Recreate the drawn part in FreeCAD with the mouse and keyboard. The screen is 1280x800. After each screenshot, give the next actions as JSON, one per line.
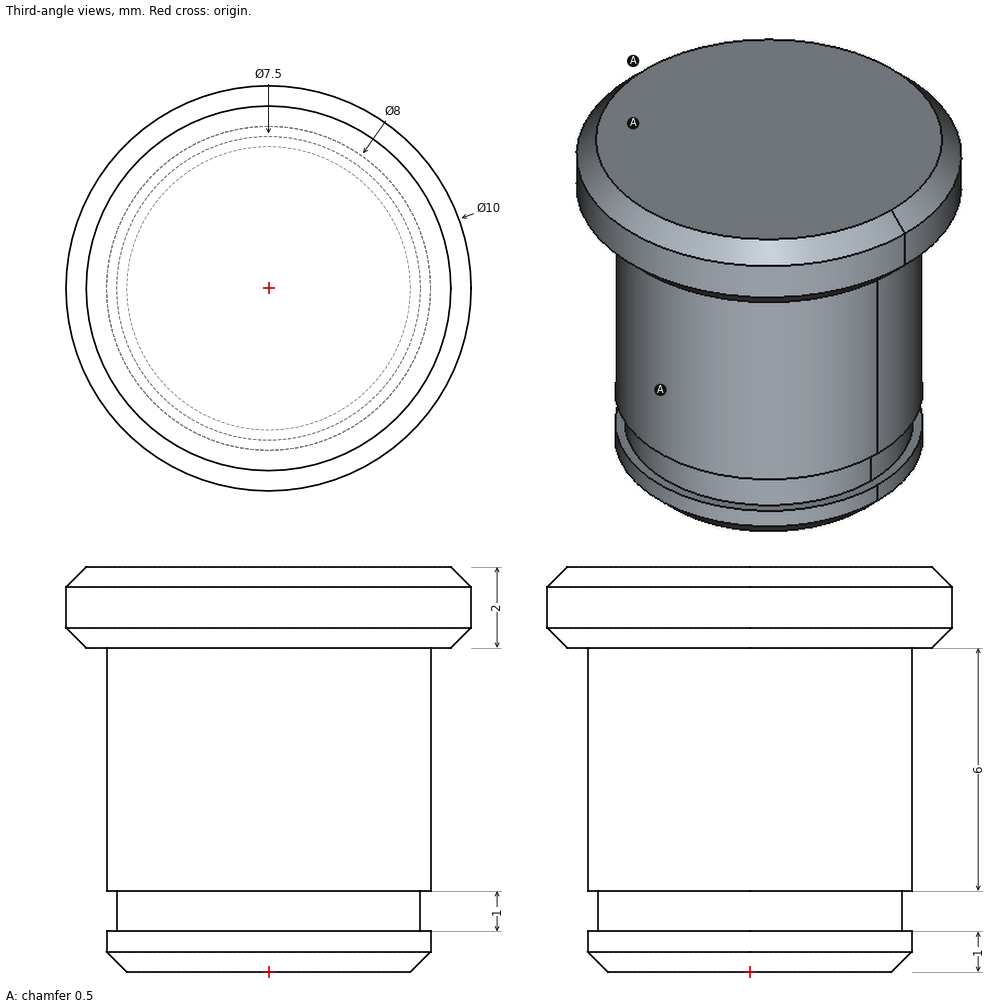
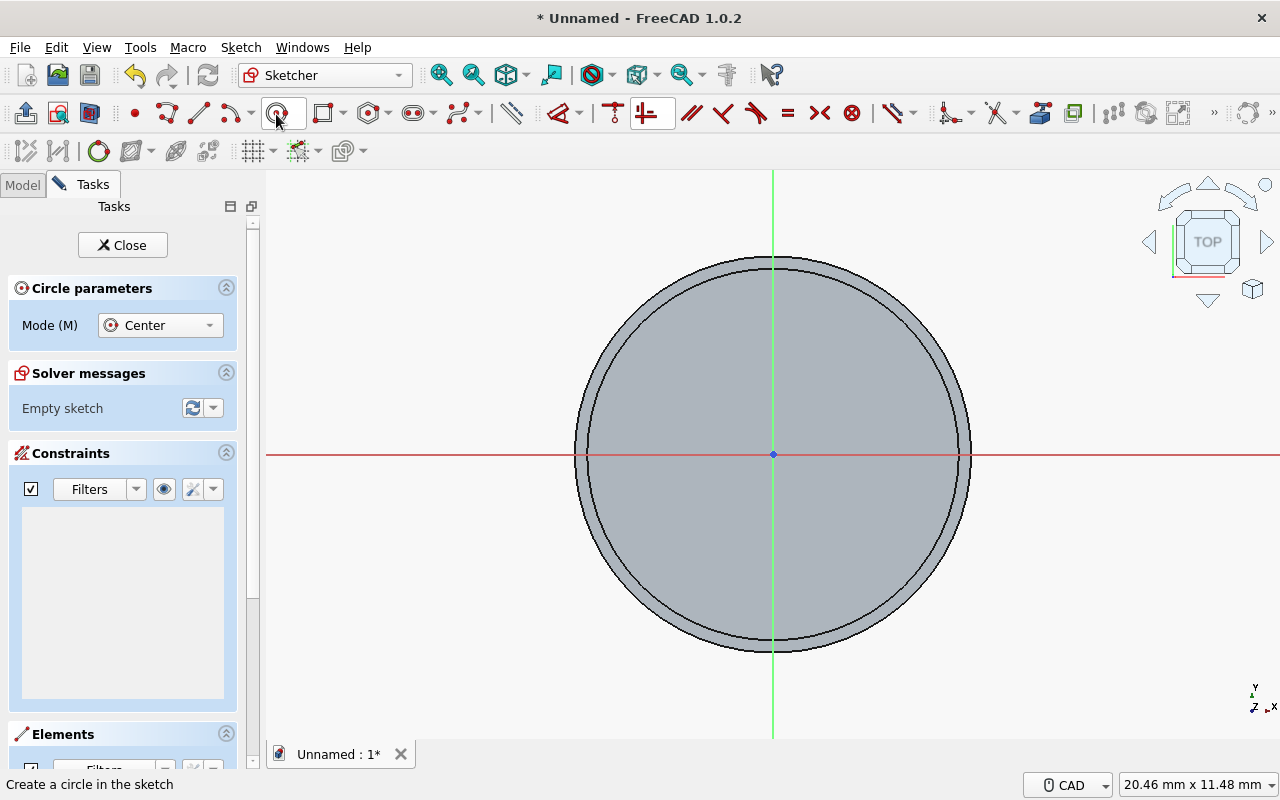
{"action": "left_click", "coordinate": [773, 454]}
{"action": "left_click", "coordinate": [913, 314]}
{"action": "key", "text": "Escape"}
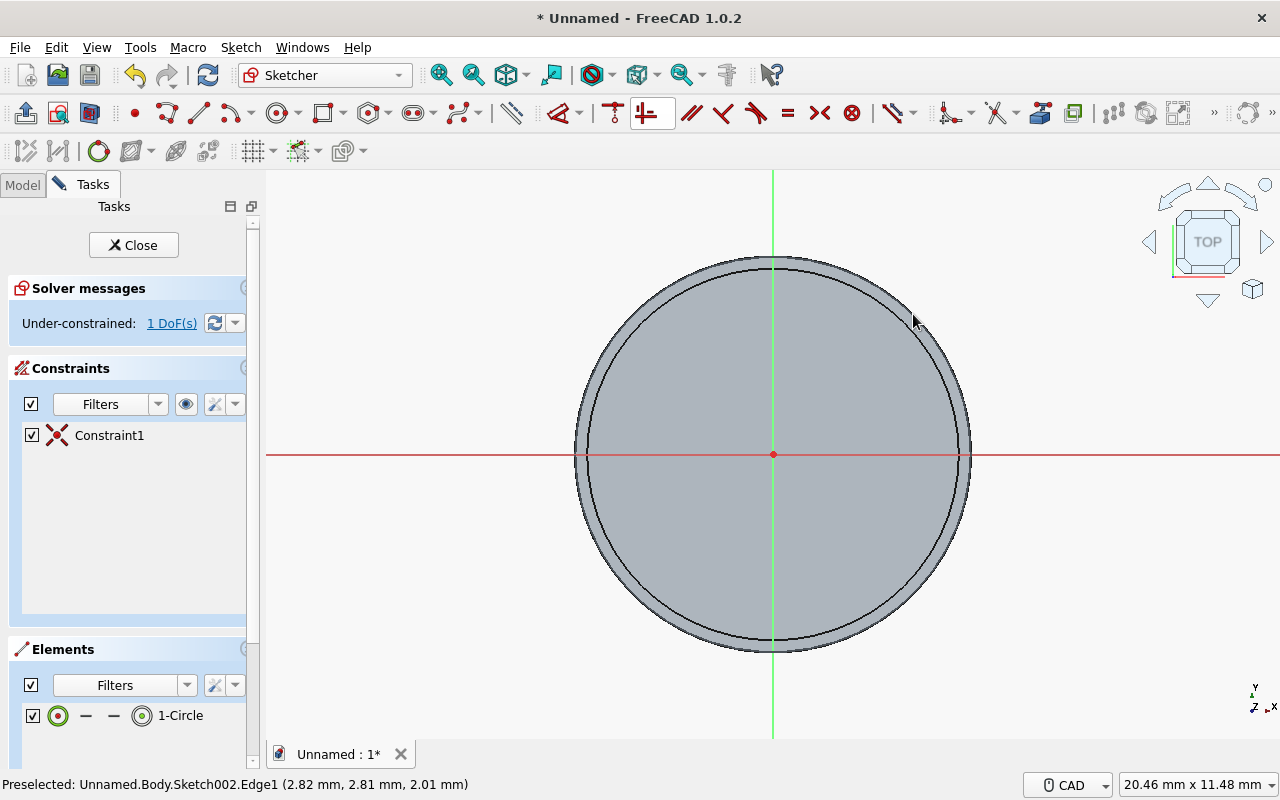
{"action": "key", "text": "d"}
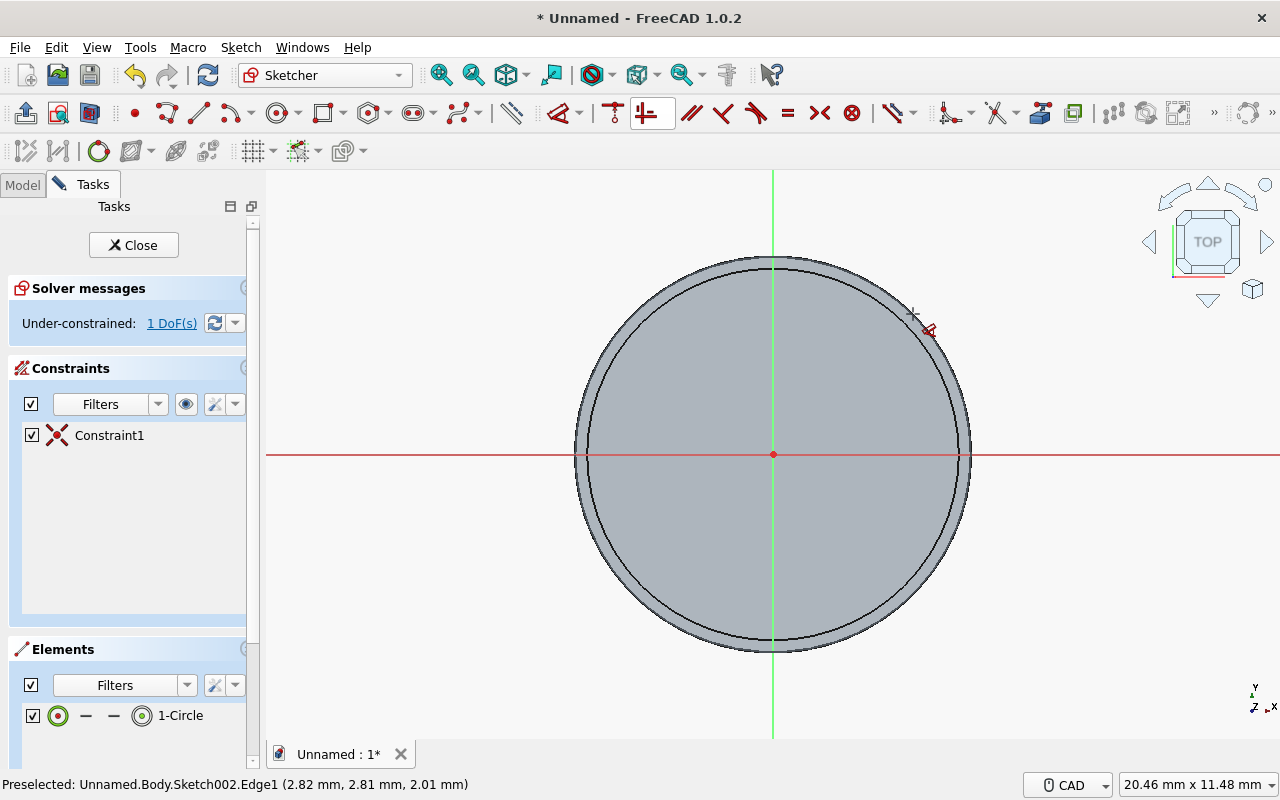
{"action": "left_click", "coordinate": [912, 314]}
{"action": "left_click", "coordinate": [935, 291]}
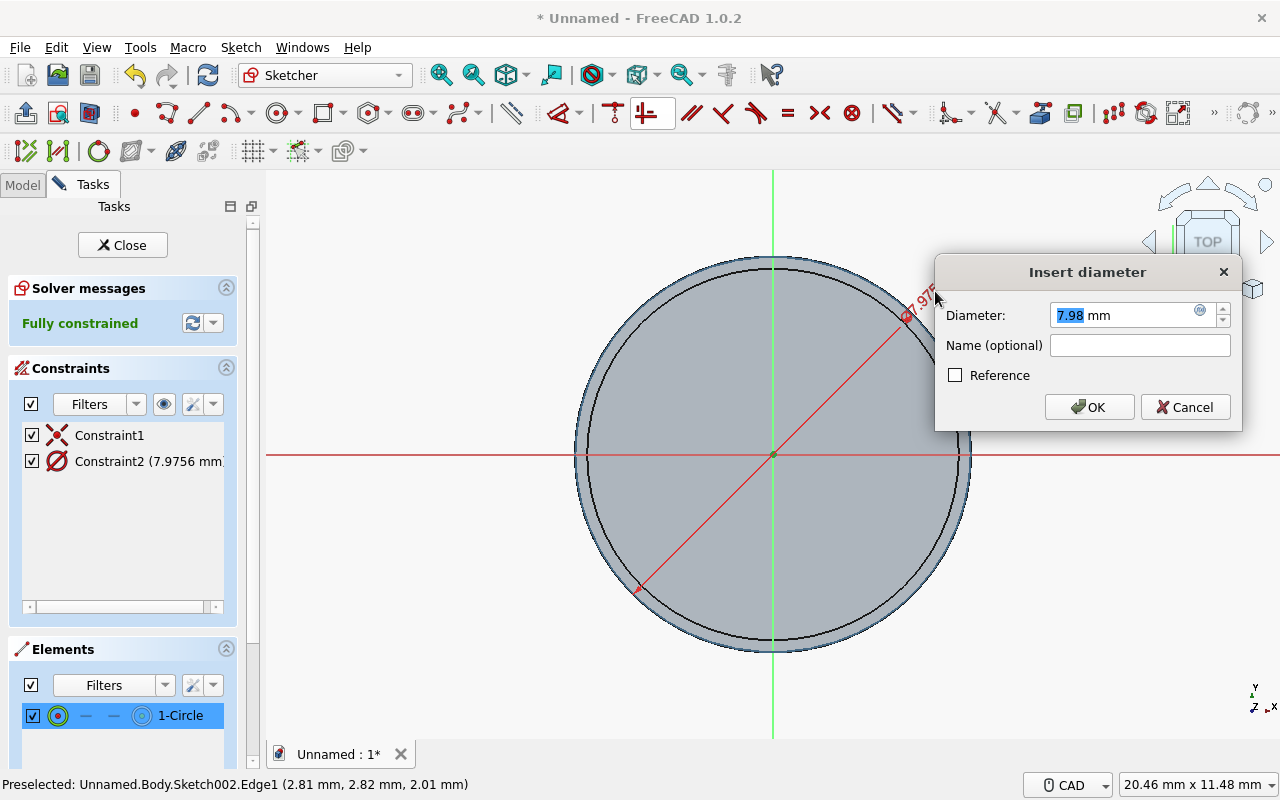
{"action": "type", "text": "8"}
{"action": "key", "text": "Return"}
{"action": "key", "text": "Escape"}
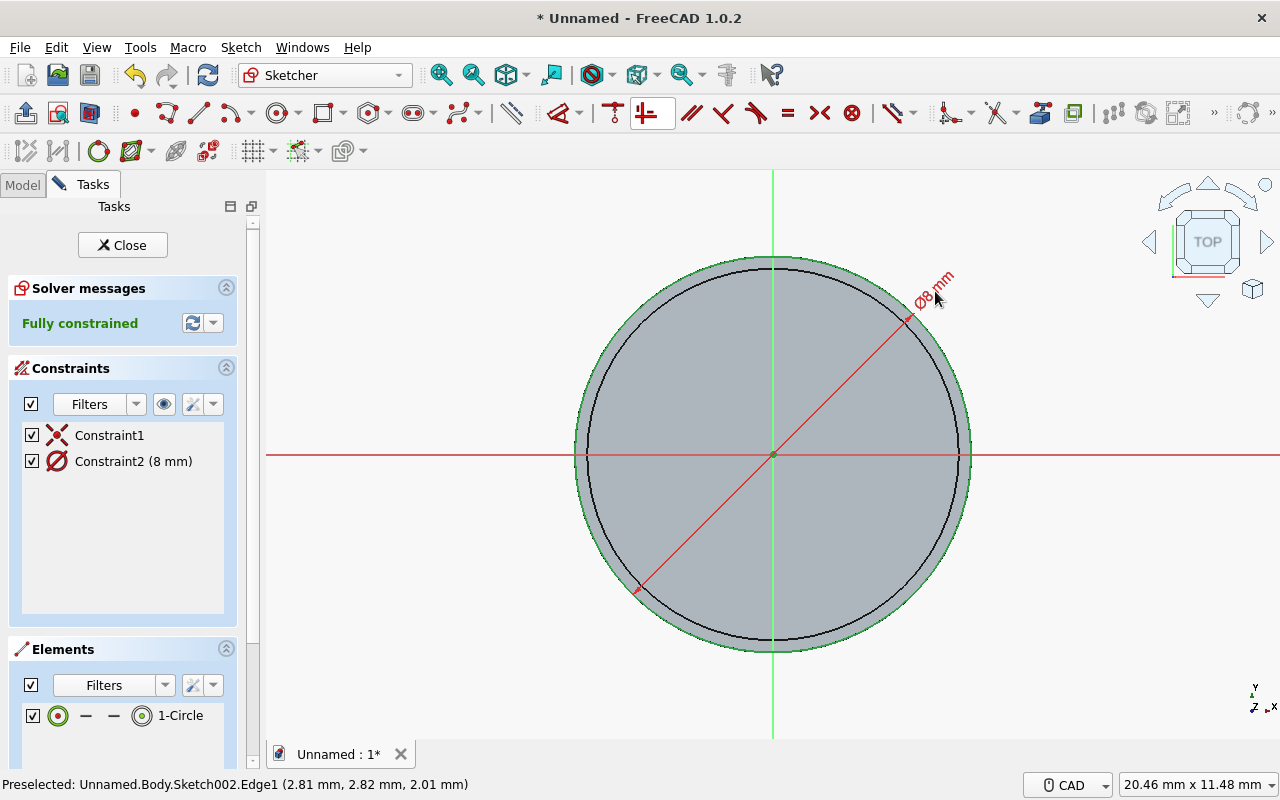
{"action": "left_click", "coordinate": [123, 245]}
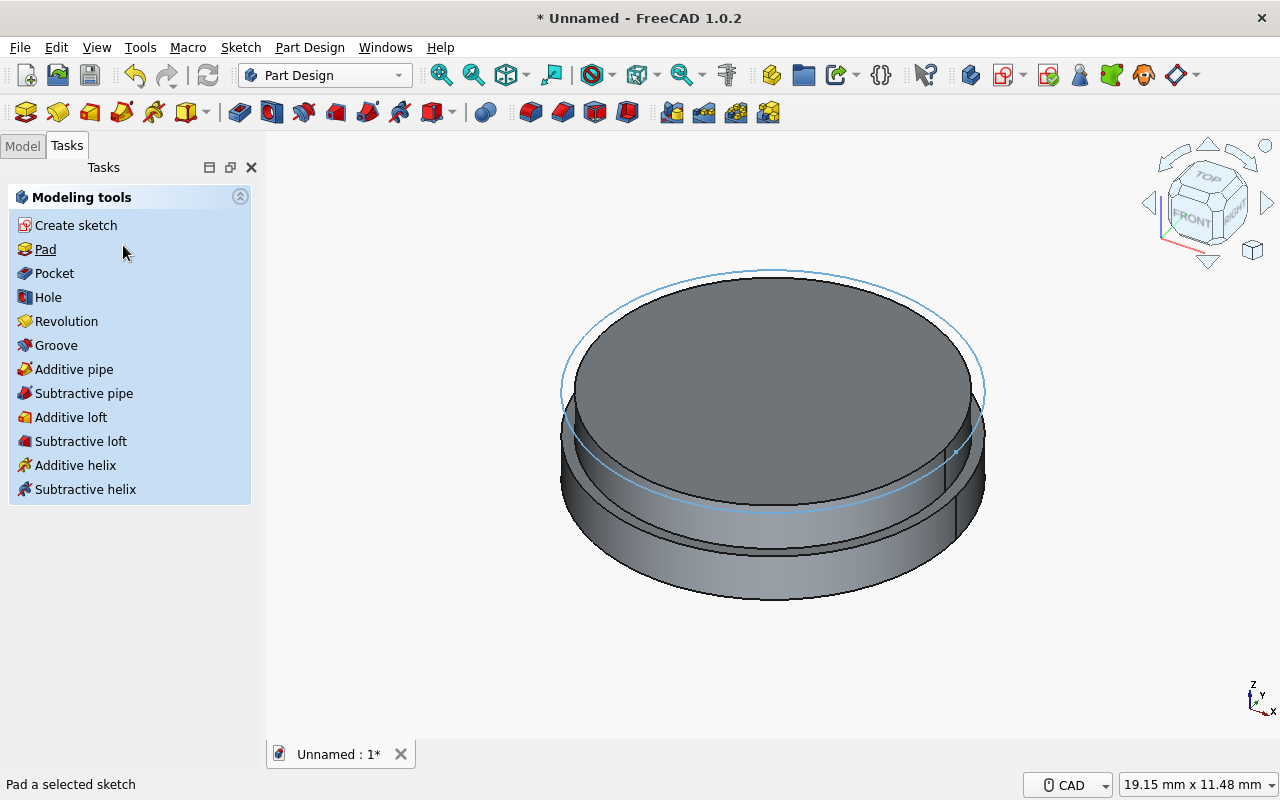
{"action": "left_click", "coordinate": [26, 112]}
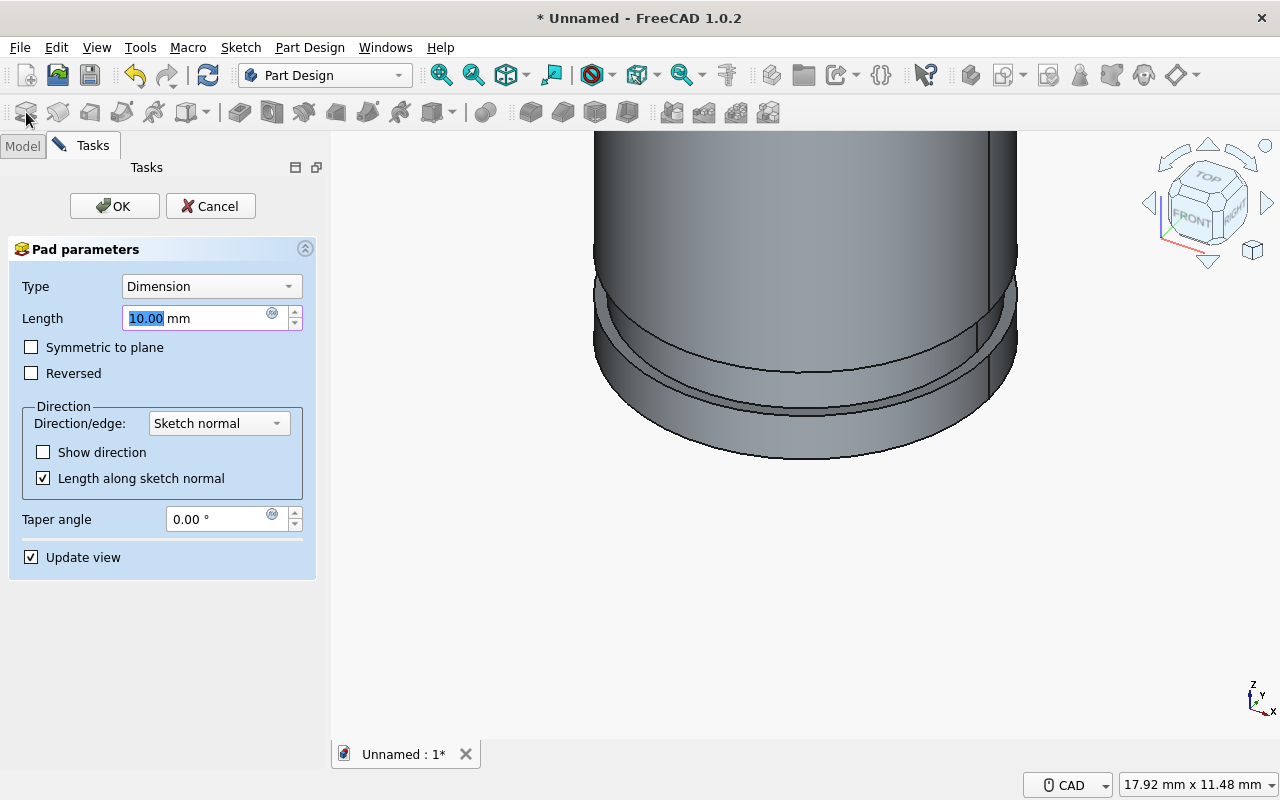
{"action": "type", "text": "6"}
{"action": "key", "text": "Tab"}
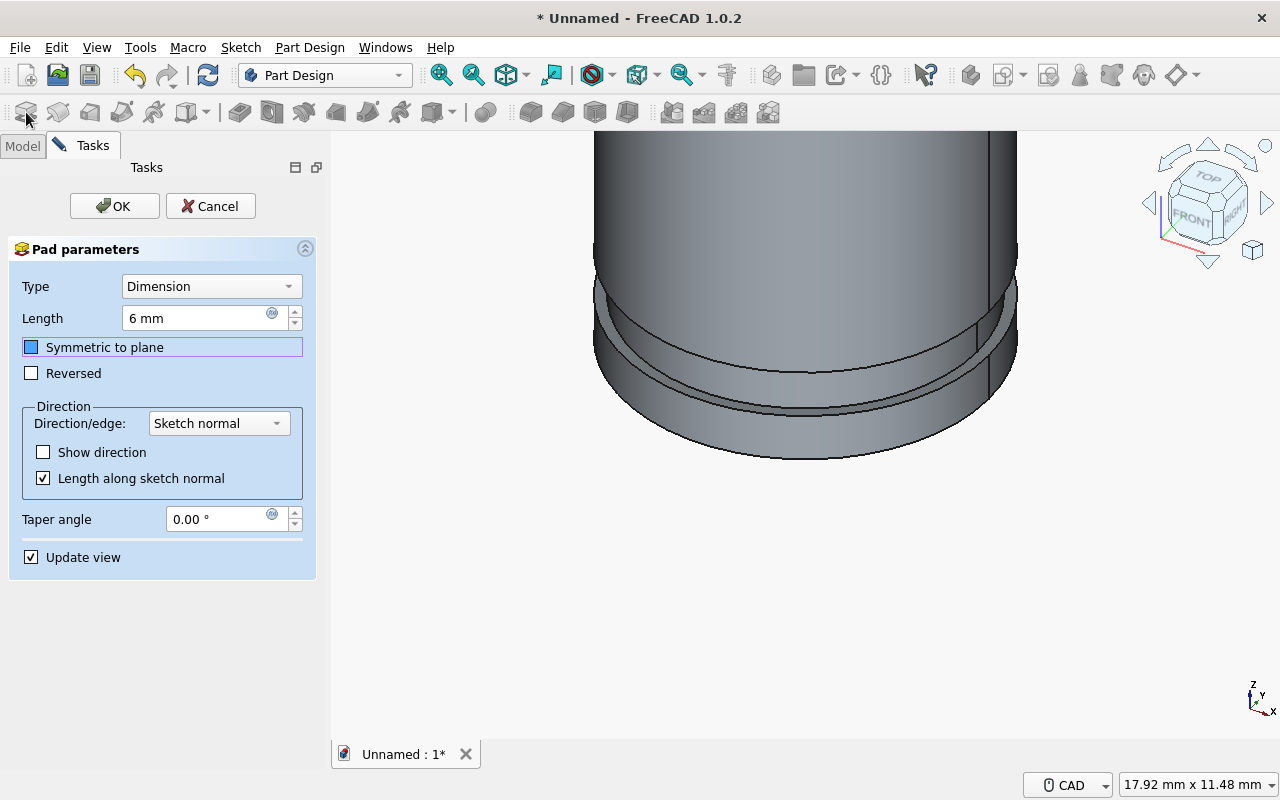
{"action": "left_click", "coordinate": [115, 206]}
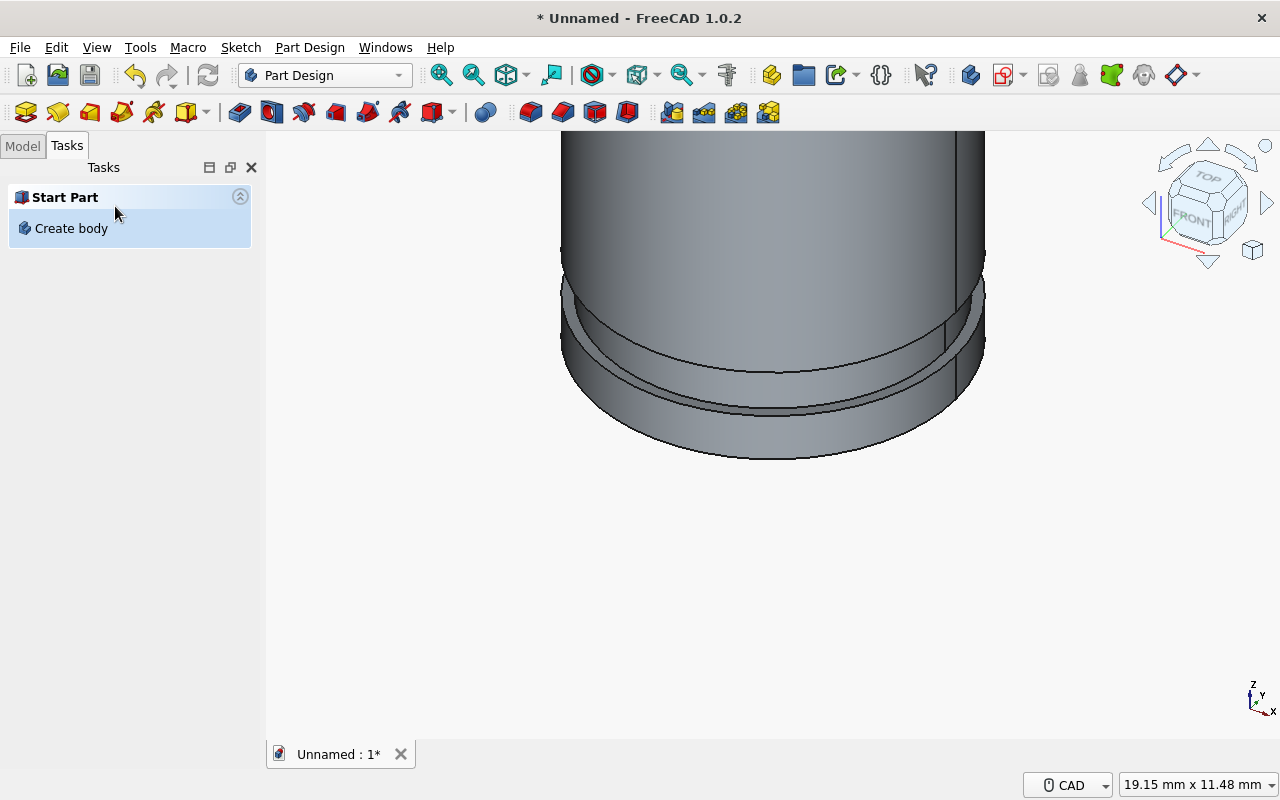
{"action": "key", "text": "v f"}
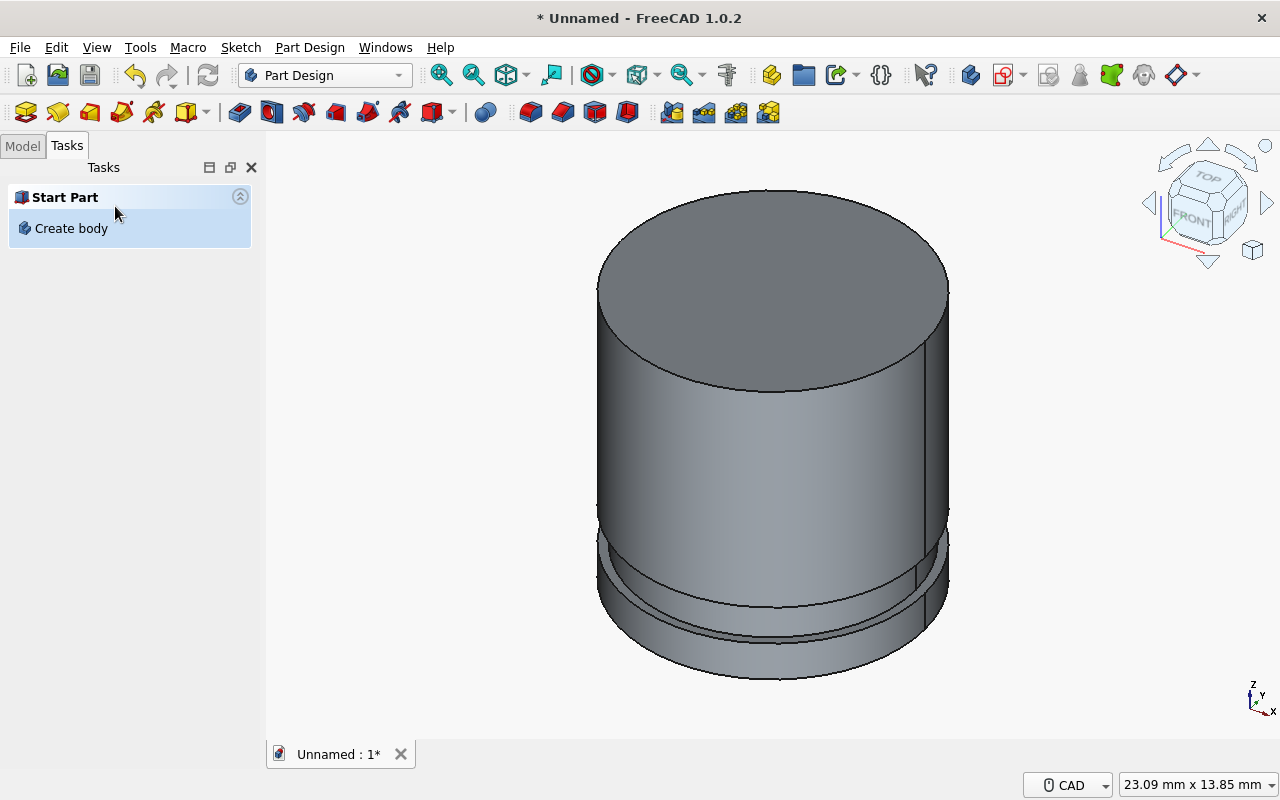
{"action": "left_click", "coordinate": [773, 290]}